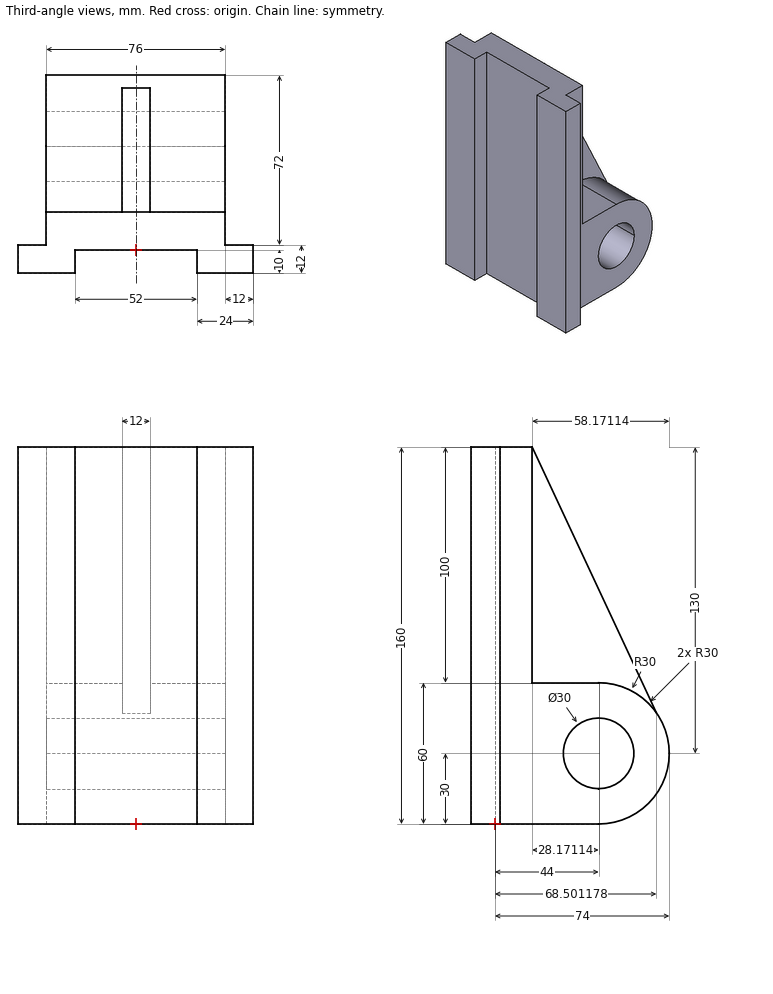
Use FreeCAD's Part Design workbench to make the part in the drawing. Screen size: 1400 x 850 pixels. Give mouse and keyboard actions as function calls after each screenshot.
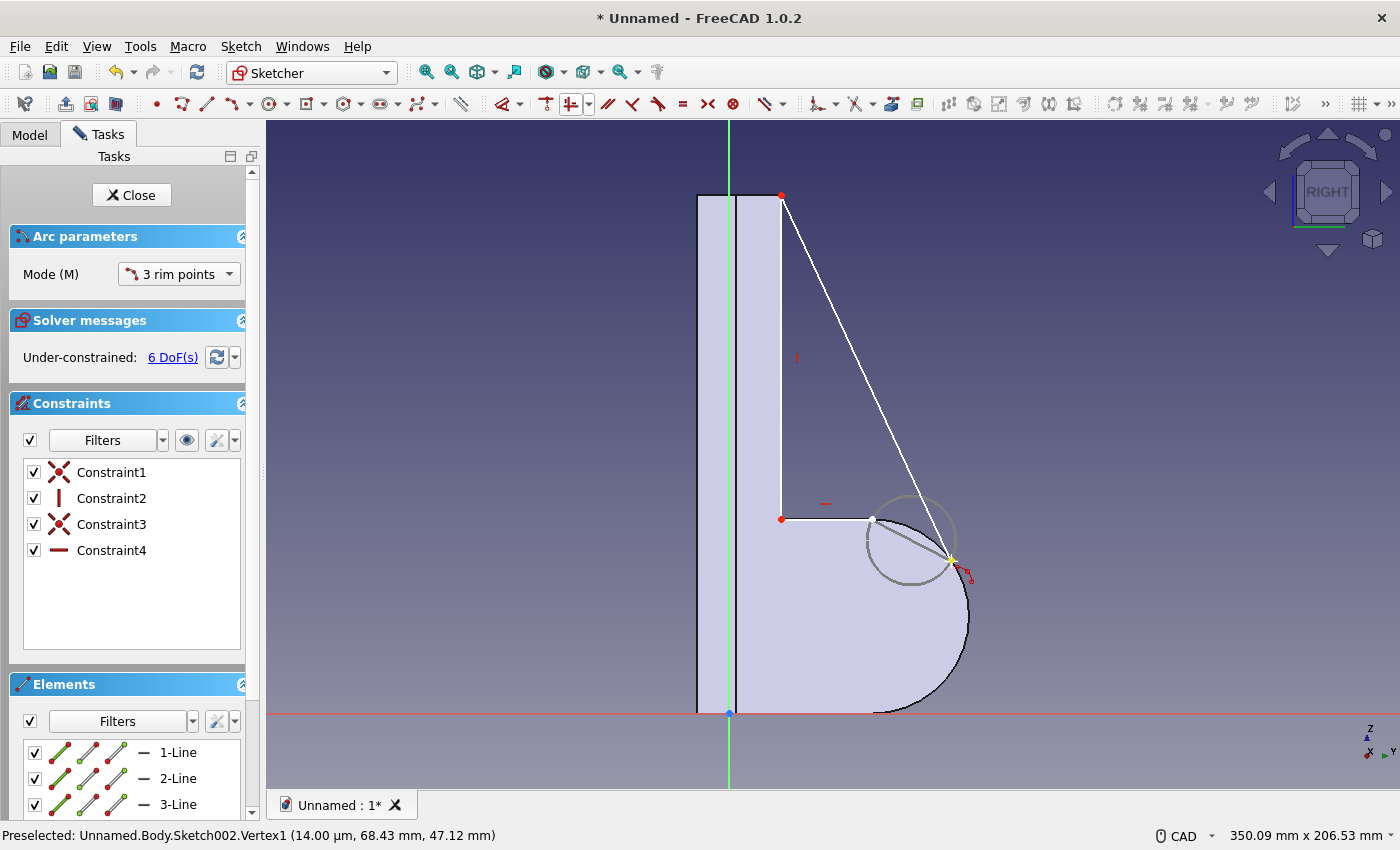
scroll(917, 530, up, 2)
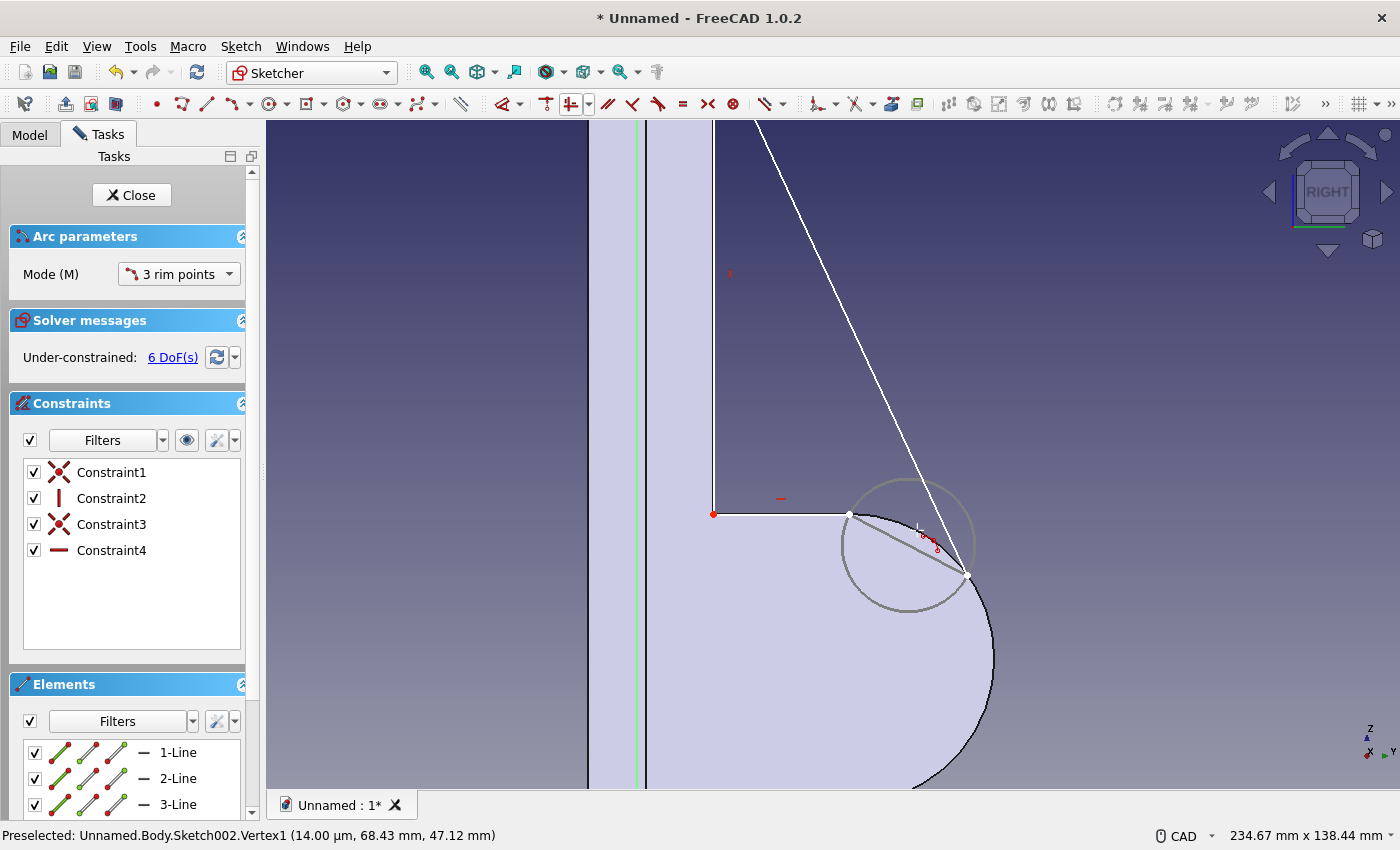
click(916, 530)
key(Escape)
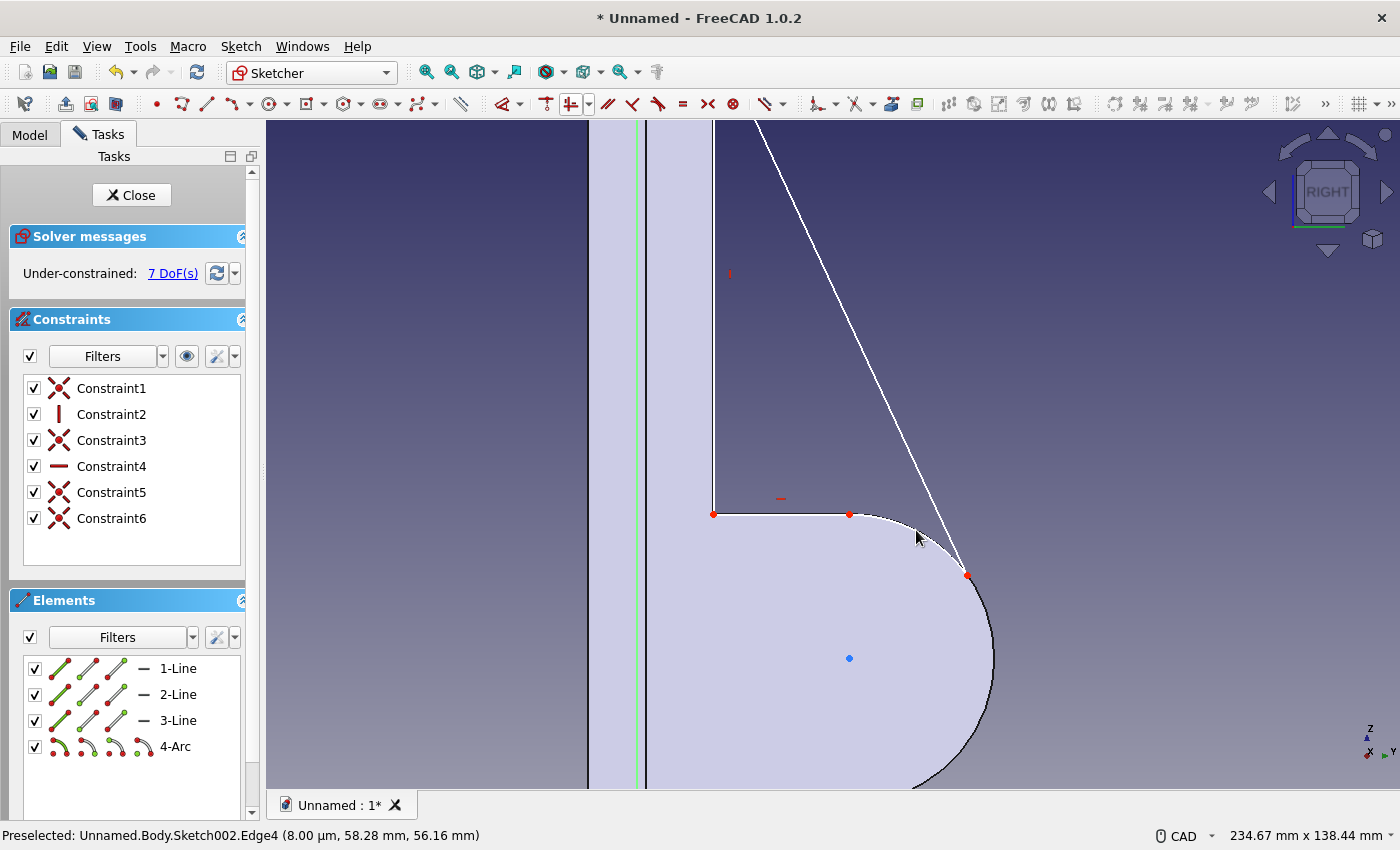
click(755, 515)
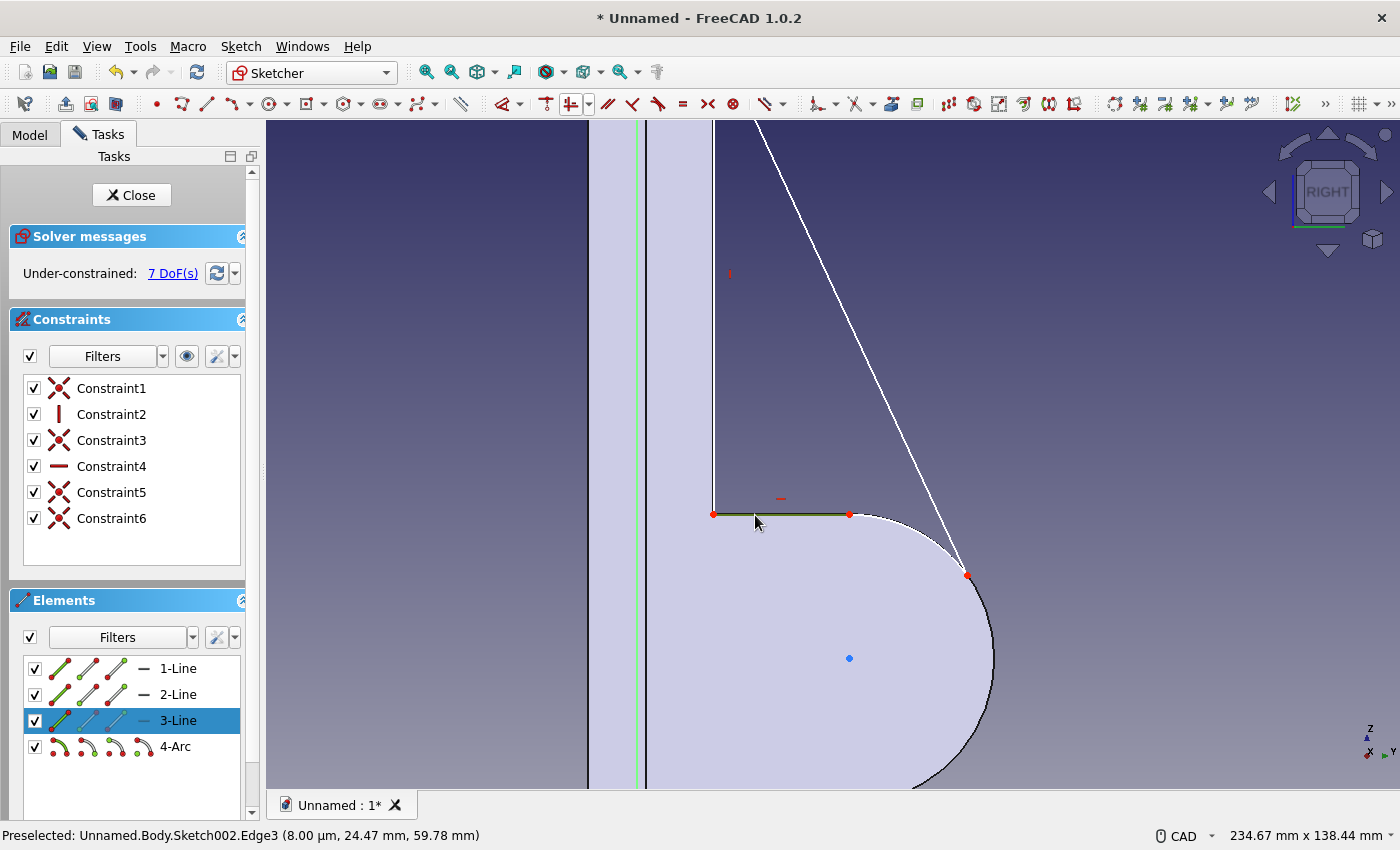
click(939, 546)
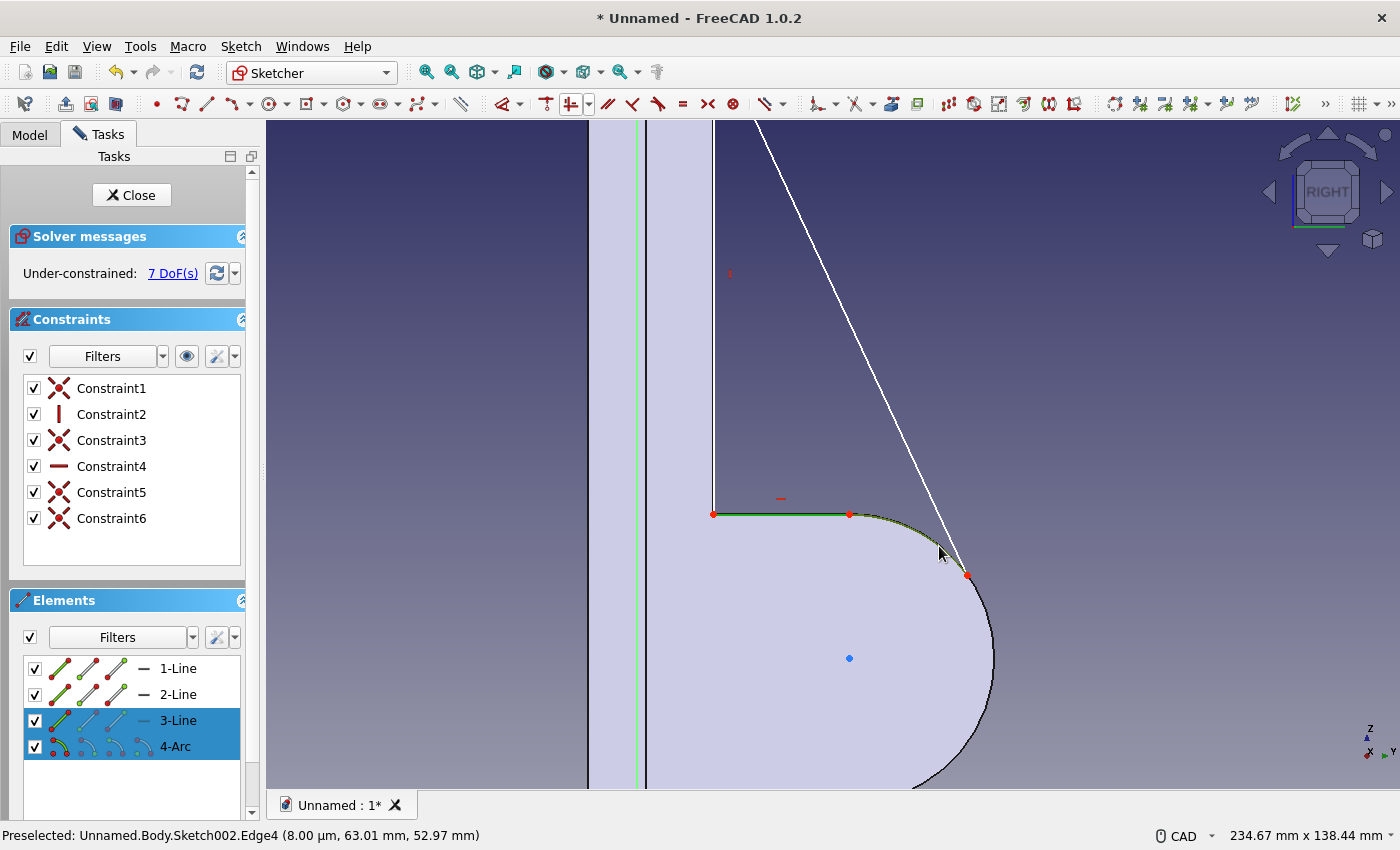
click(658, 104)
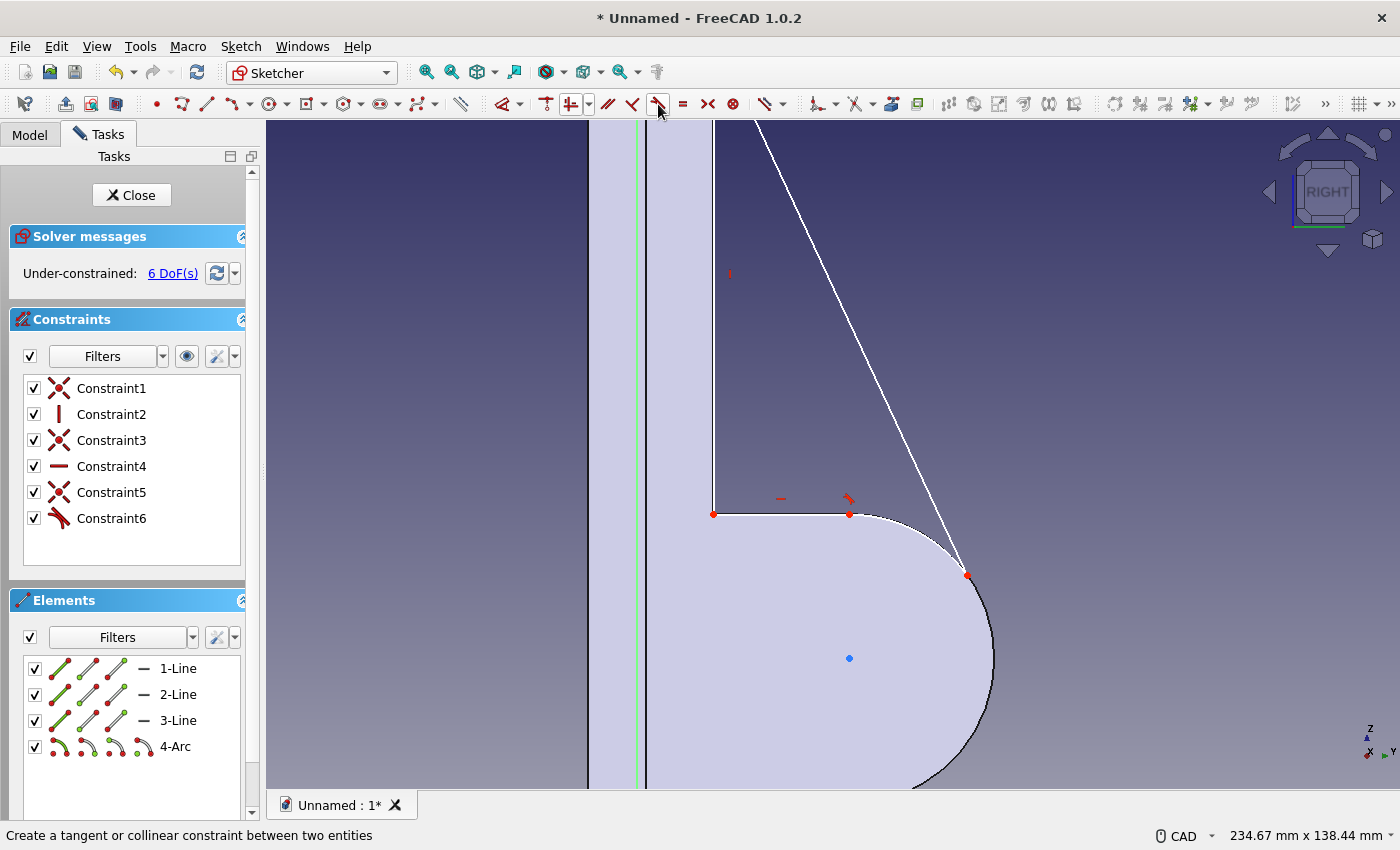
click(502, 104)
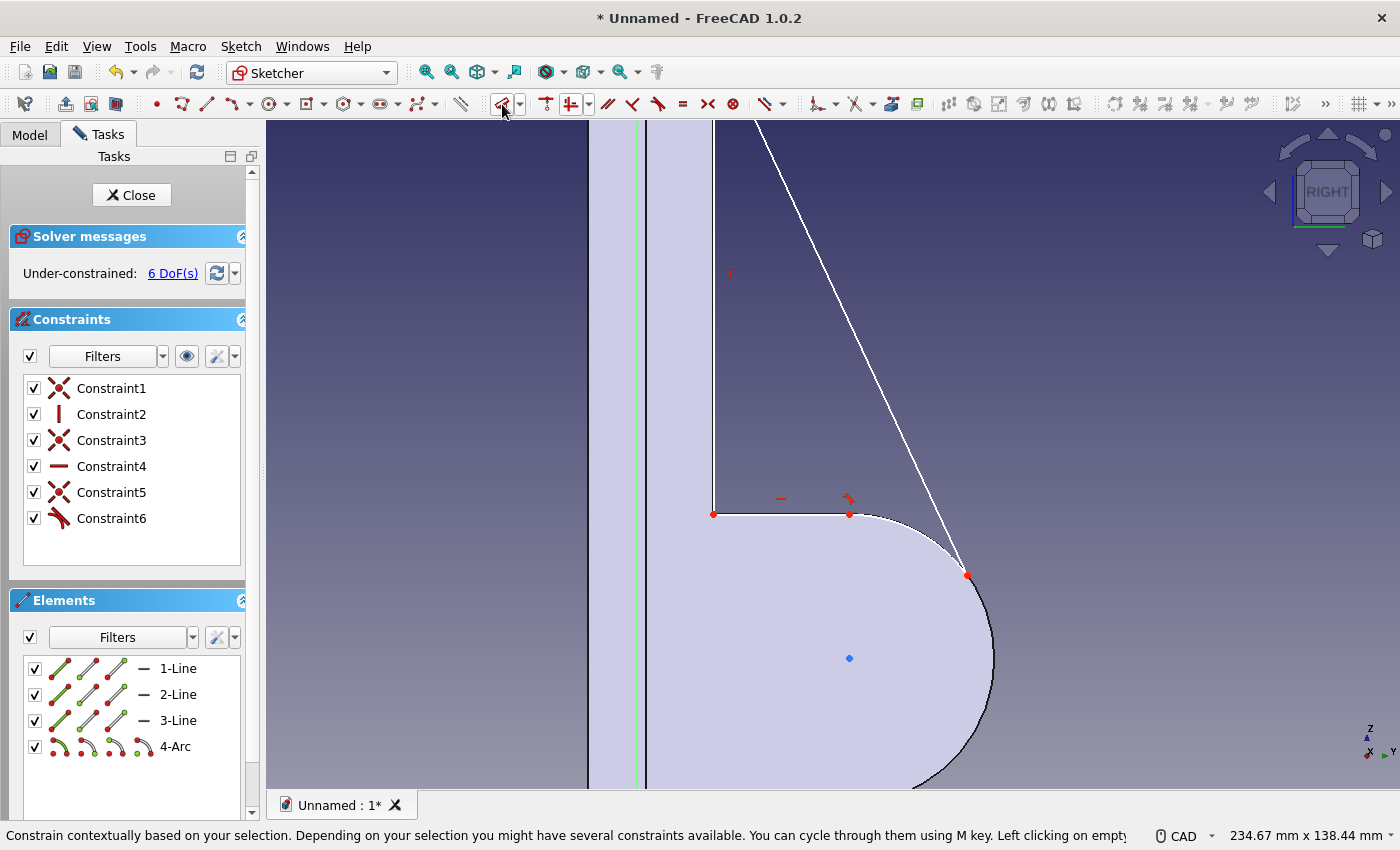
click(939, 546)
click(959, 521)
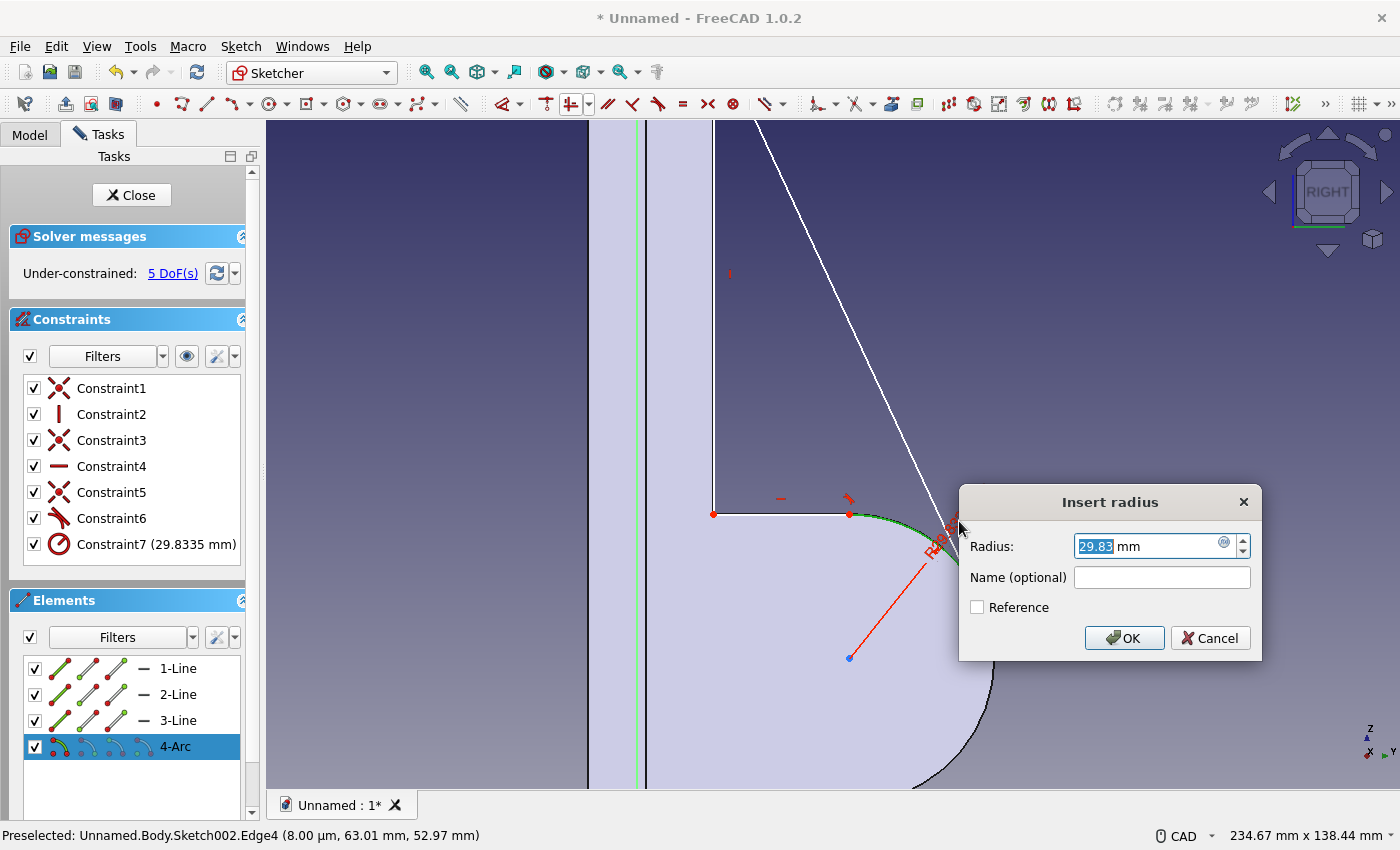
text(30)
key(Return)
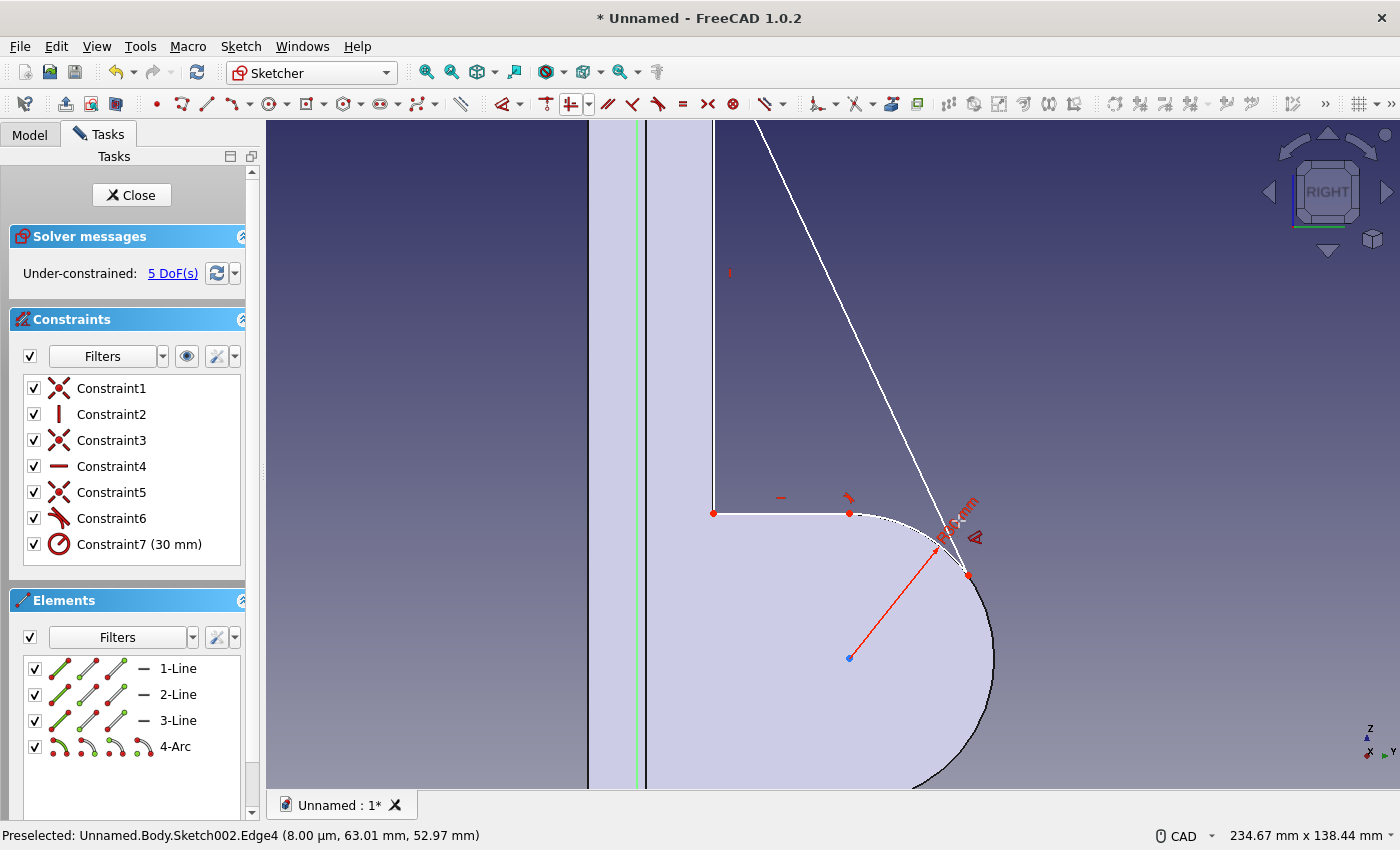
click(714, 176)
click(680, 331)